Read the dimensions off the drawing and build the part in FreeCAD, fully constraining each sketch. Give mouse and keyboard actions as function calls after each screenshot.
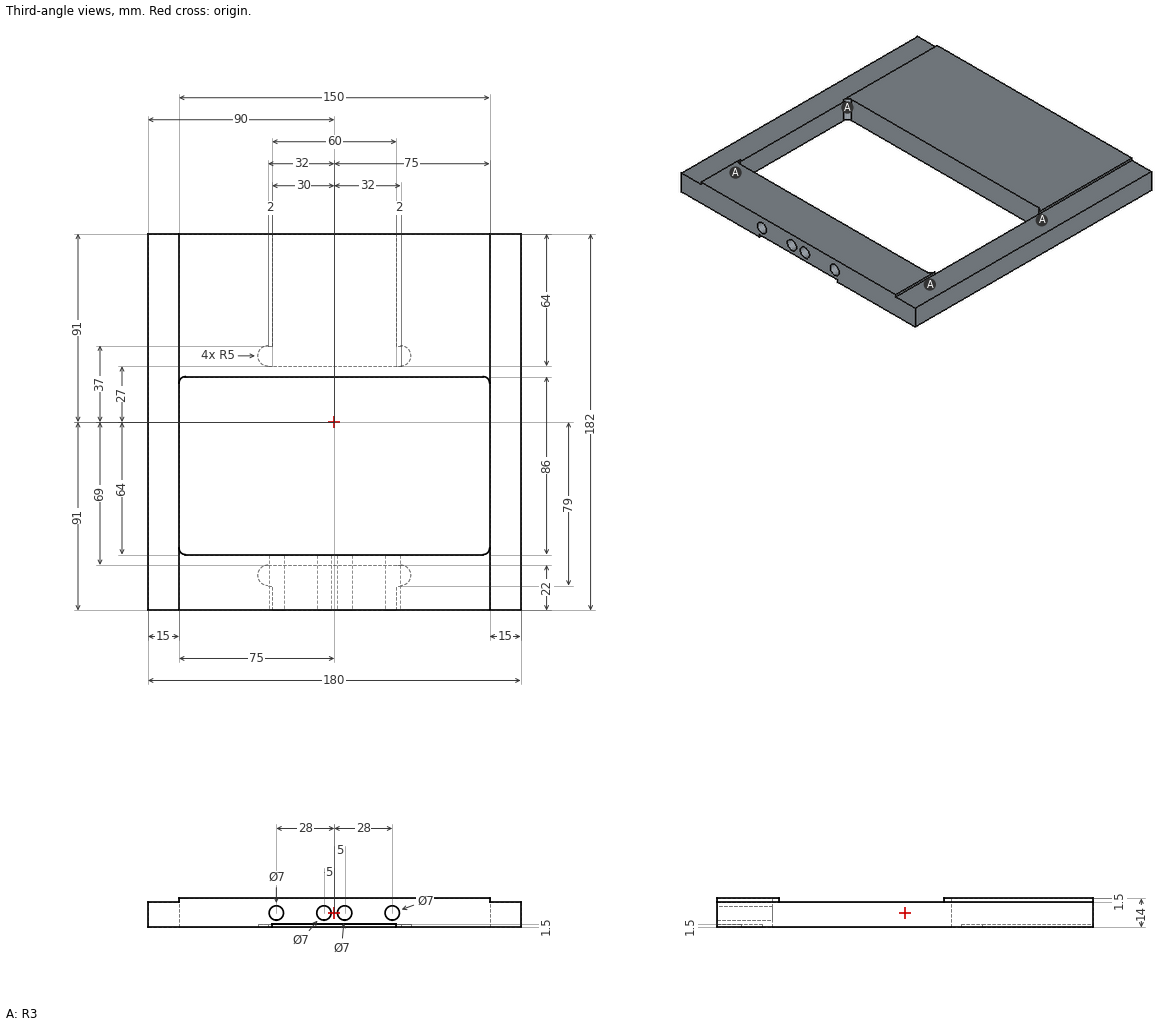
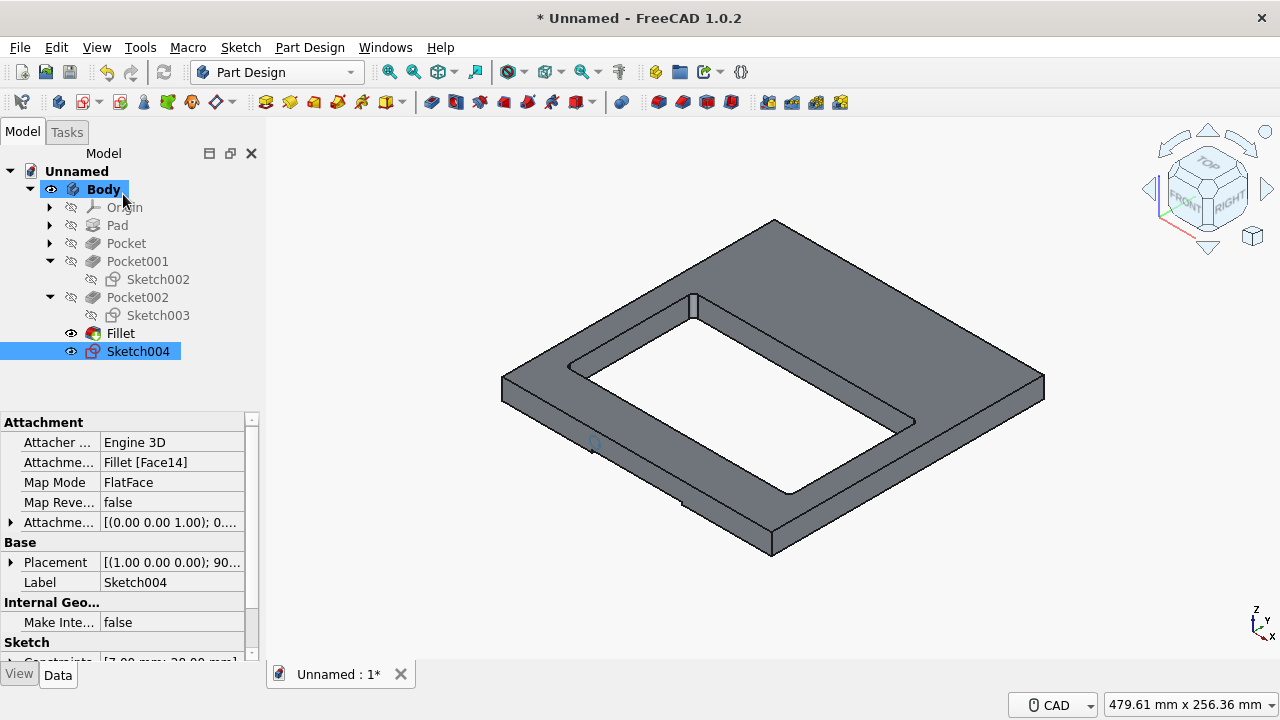
click(432, 102)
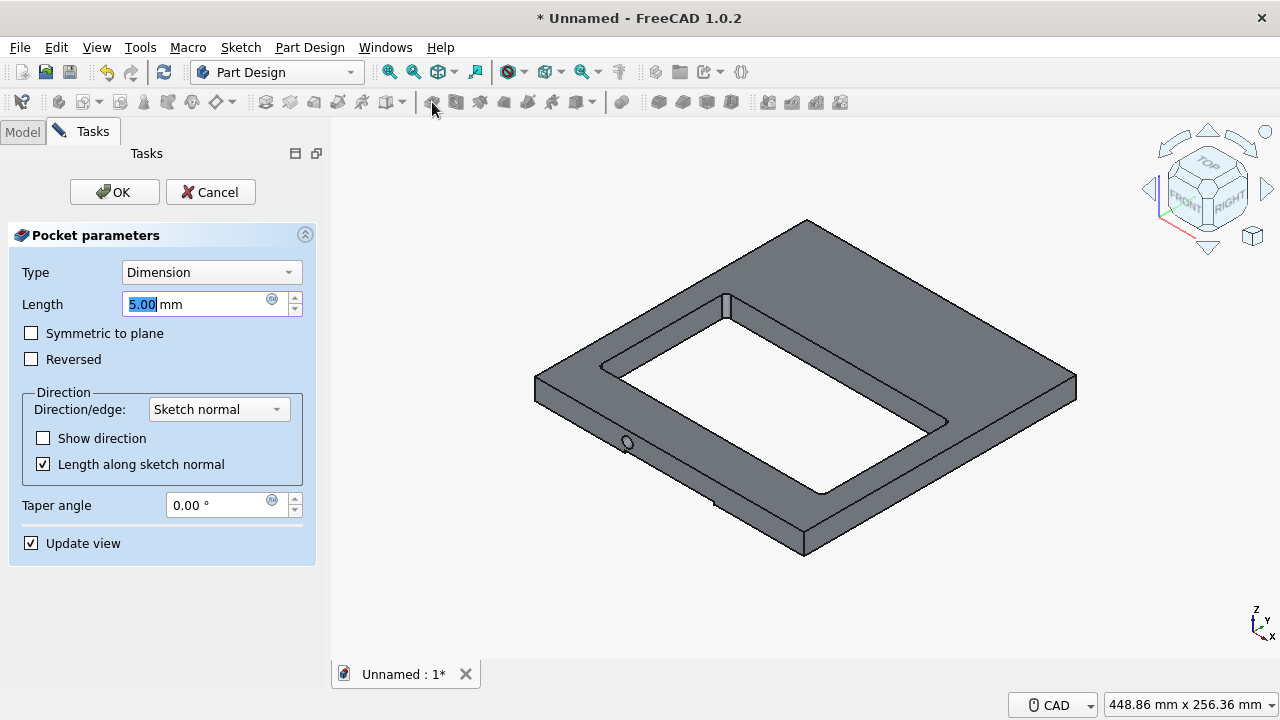
click(212, 272)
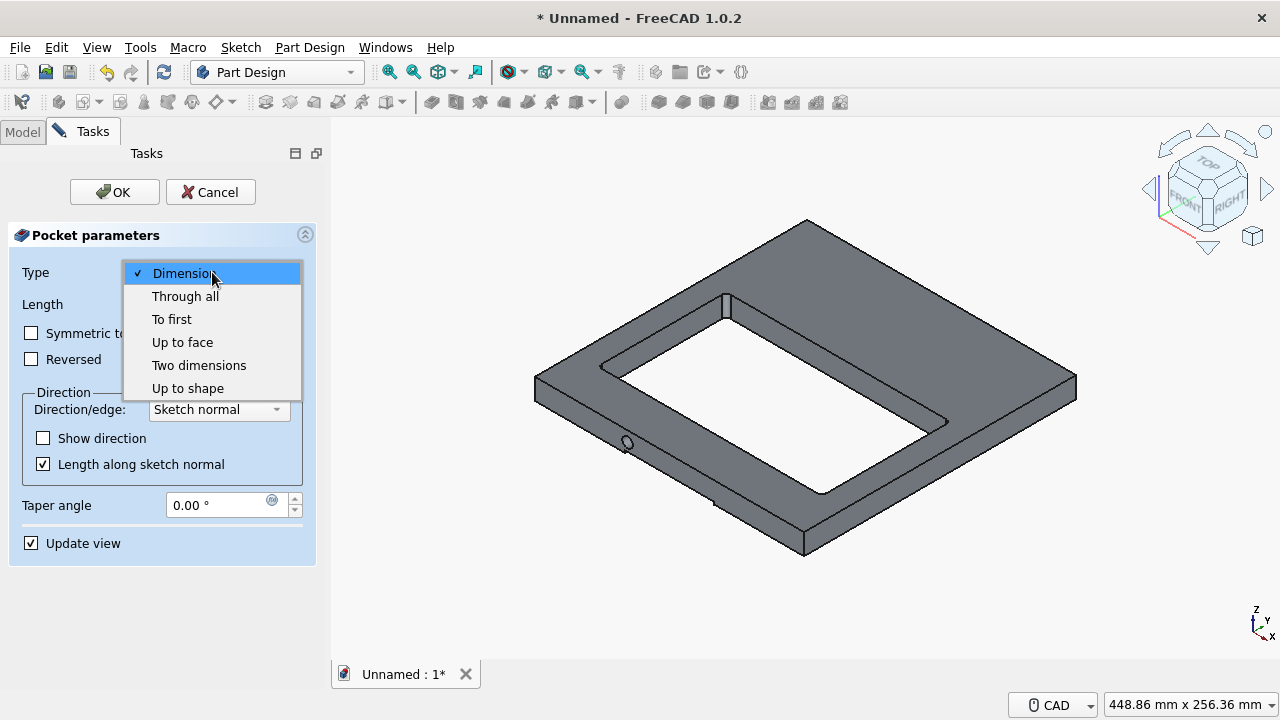
click(212, 320)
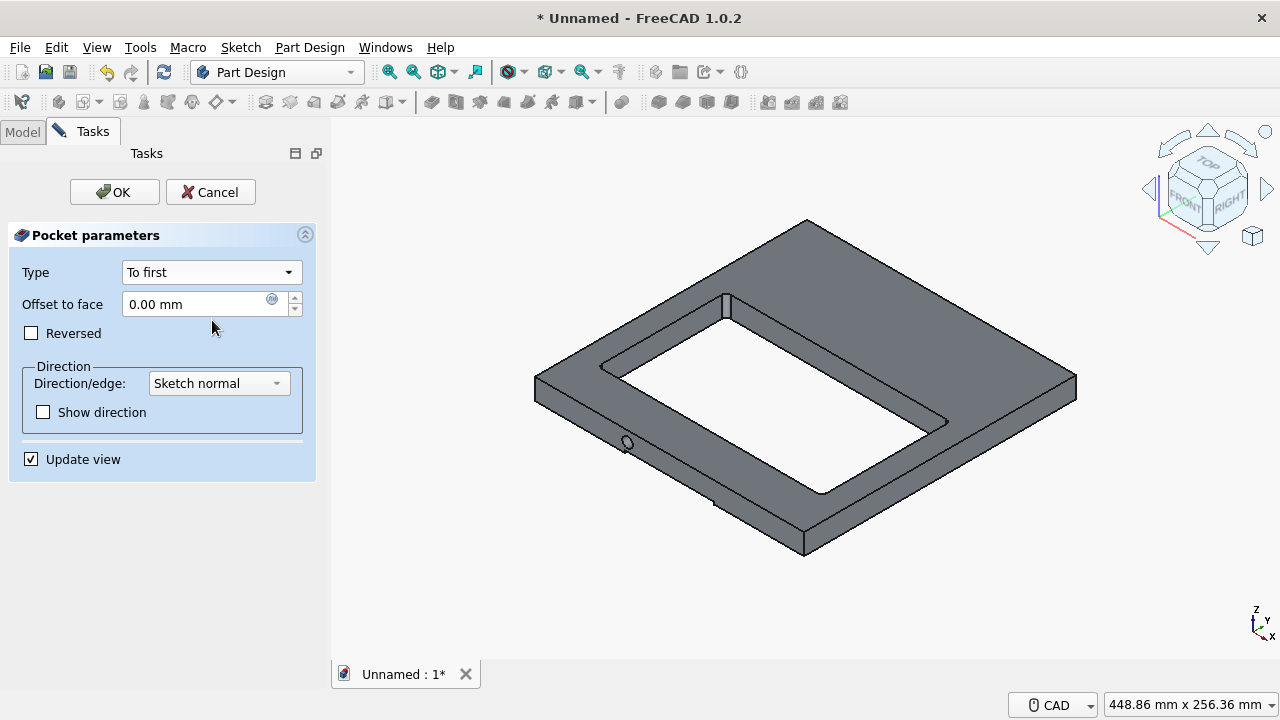
click(115, 192)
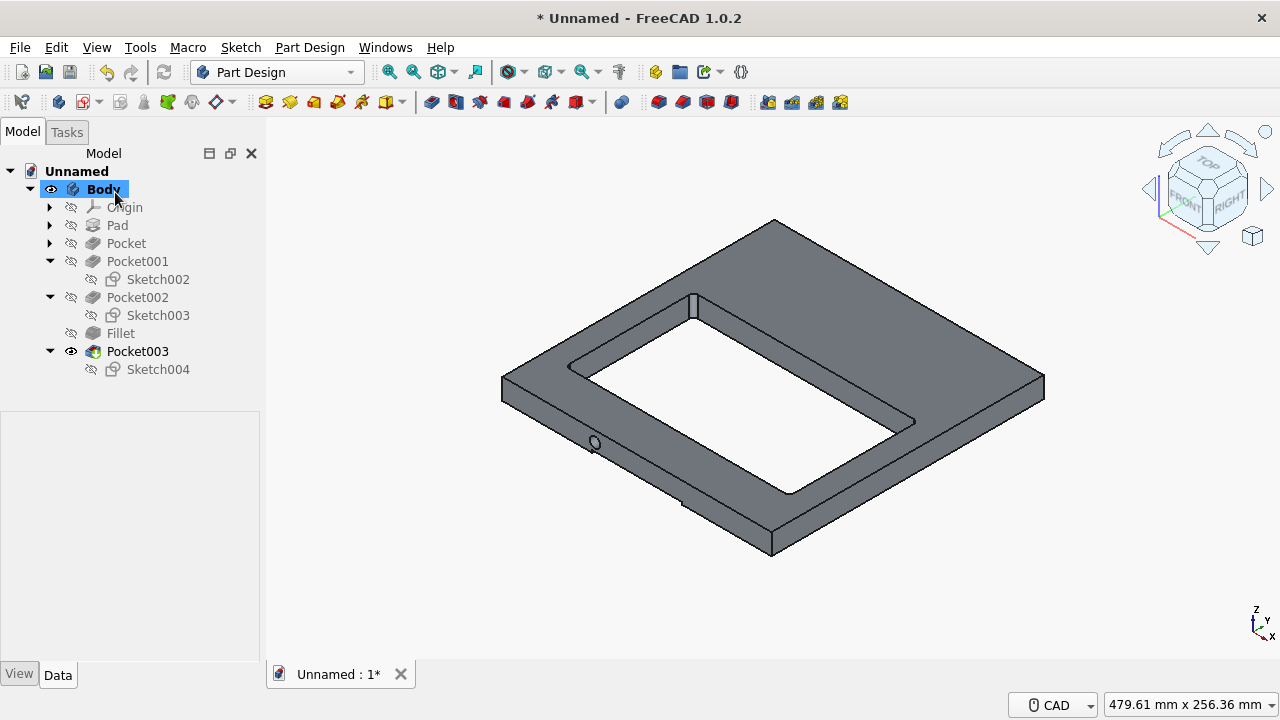
click(752, 532)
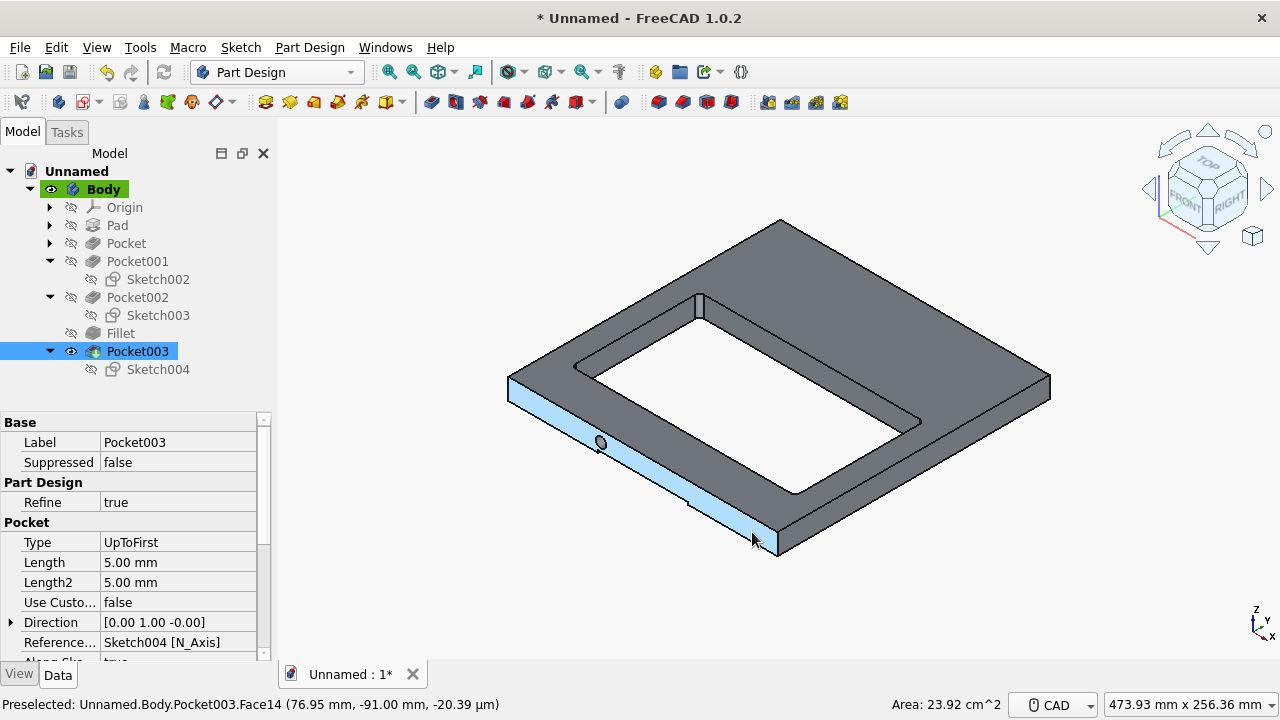
click(84, 102)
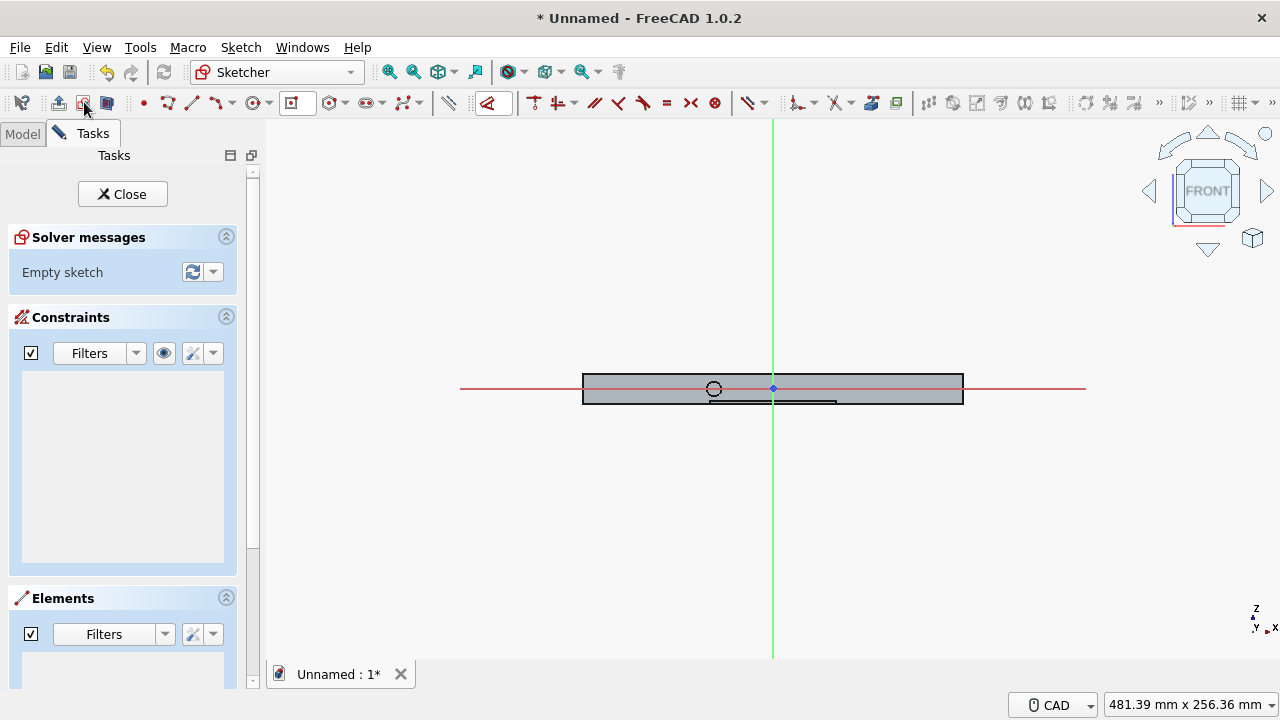
scroll(839, 389, up, 15)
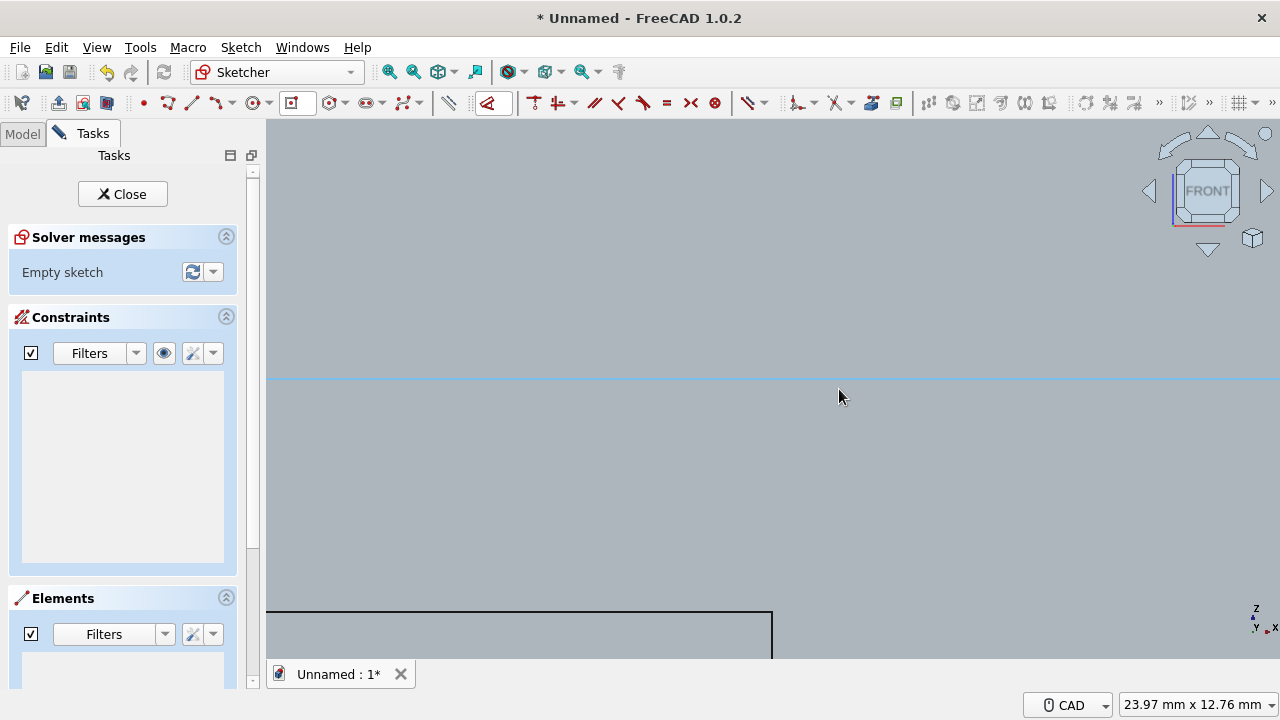
key(g)
key(c)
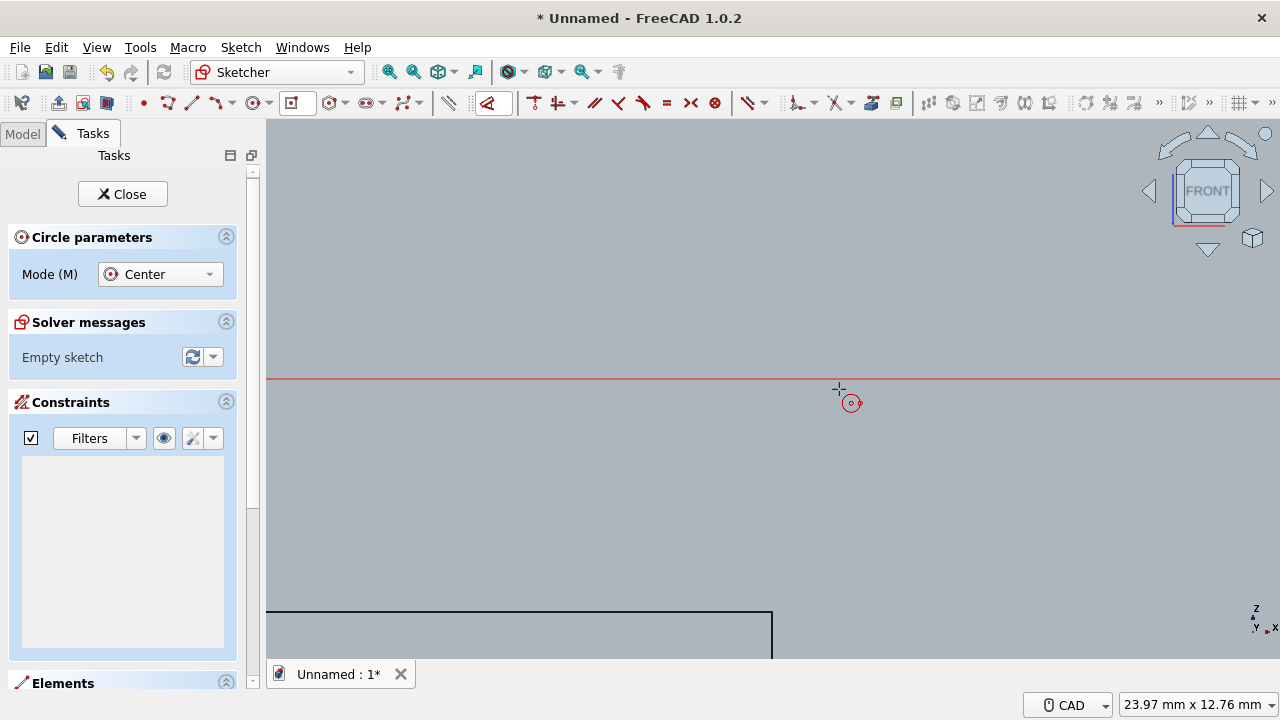
click(687, 379)
move(792, 275)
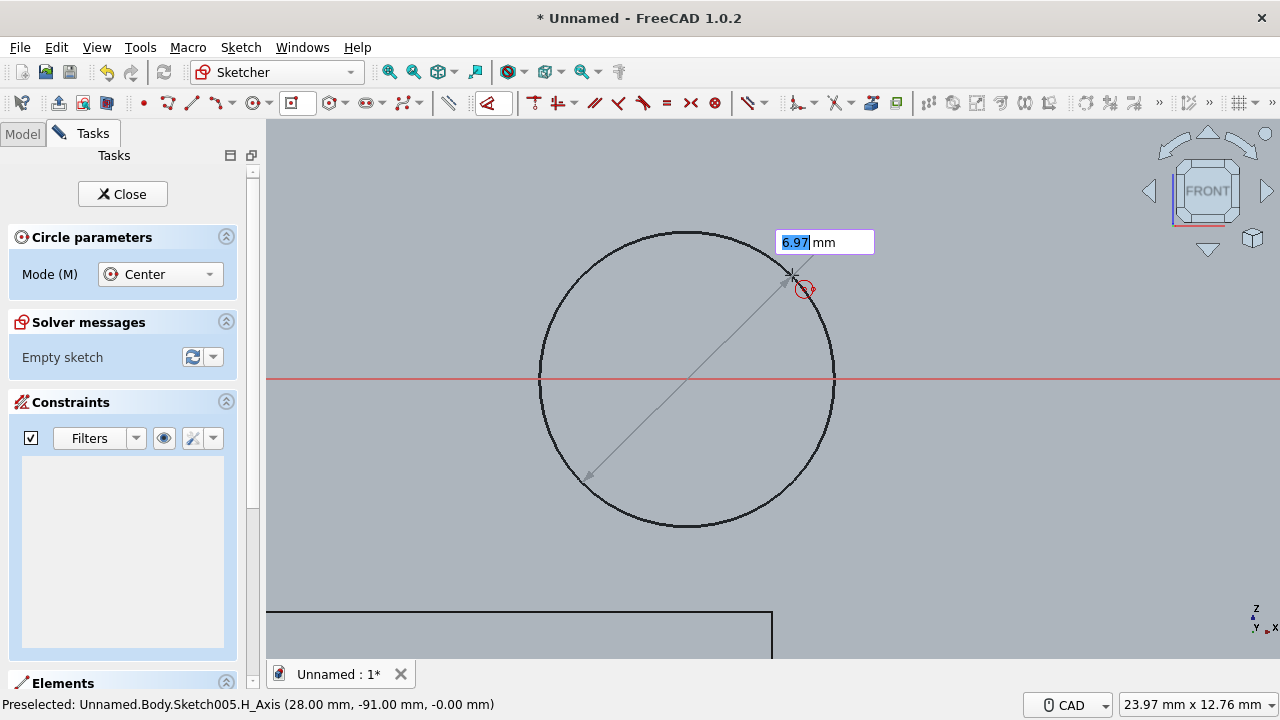
text(7)
key(Return)
key(Escape)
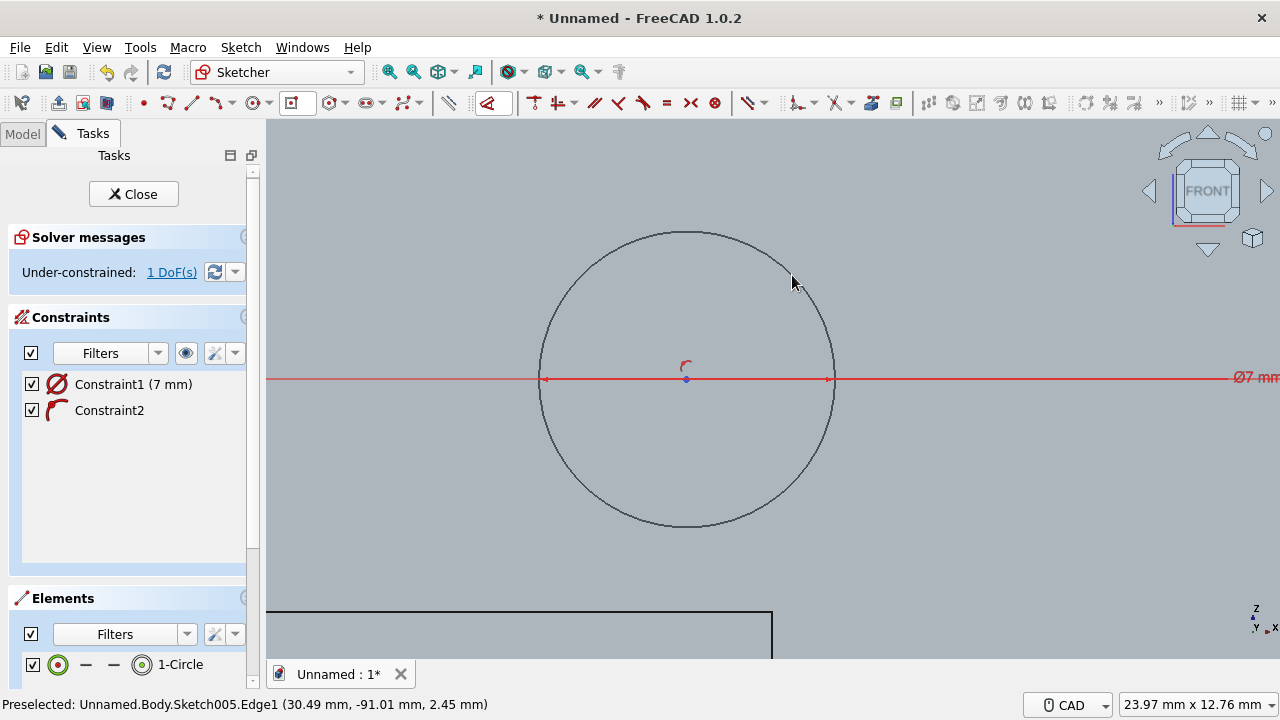
click(687, 379)